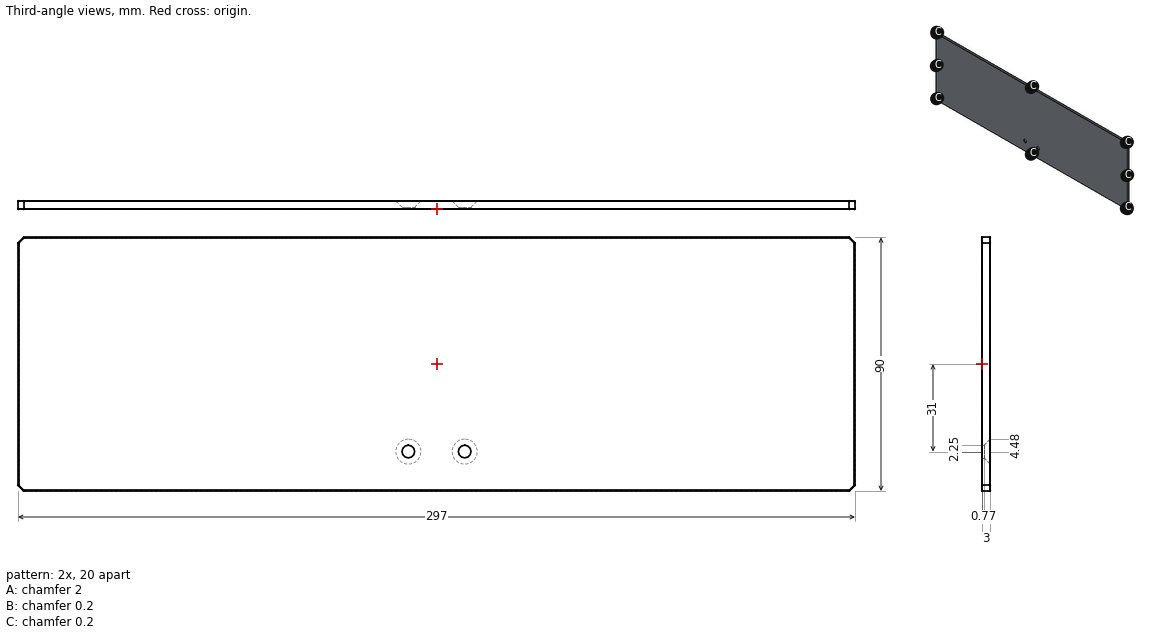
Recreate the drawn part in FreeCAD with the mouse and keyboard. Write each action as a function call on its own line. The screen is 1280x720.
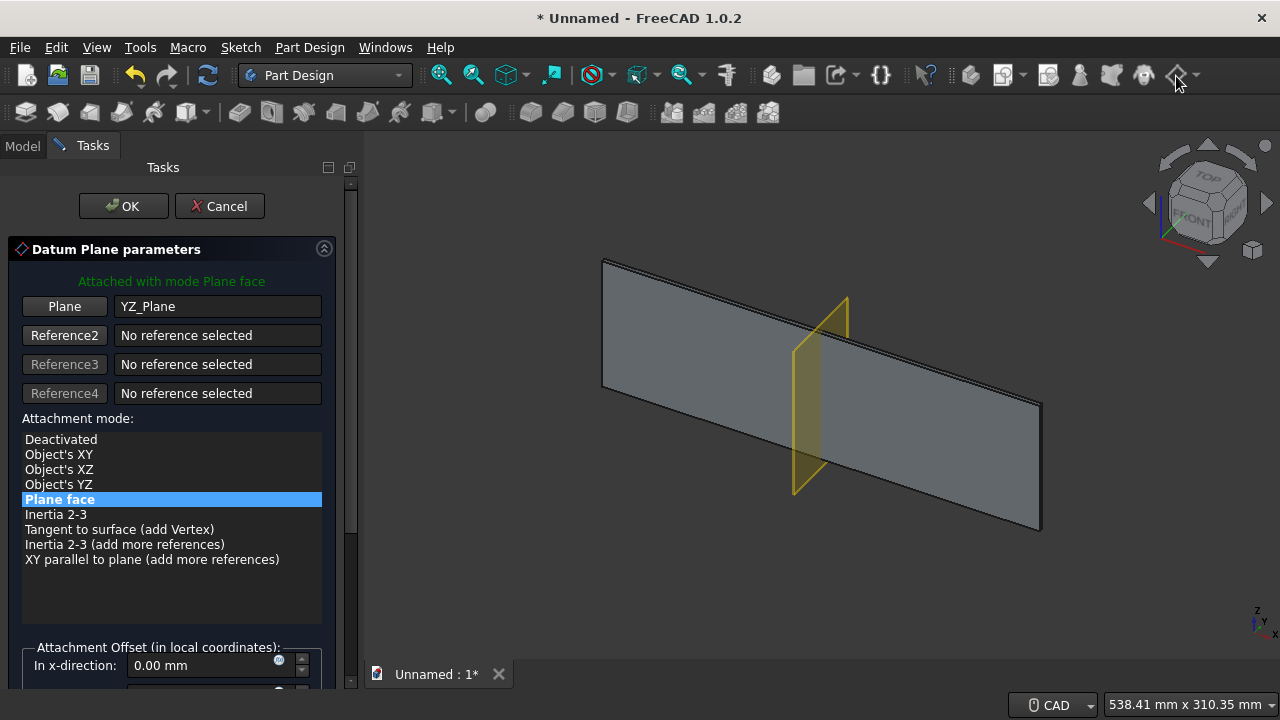
scroll(351, 432, down, 2)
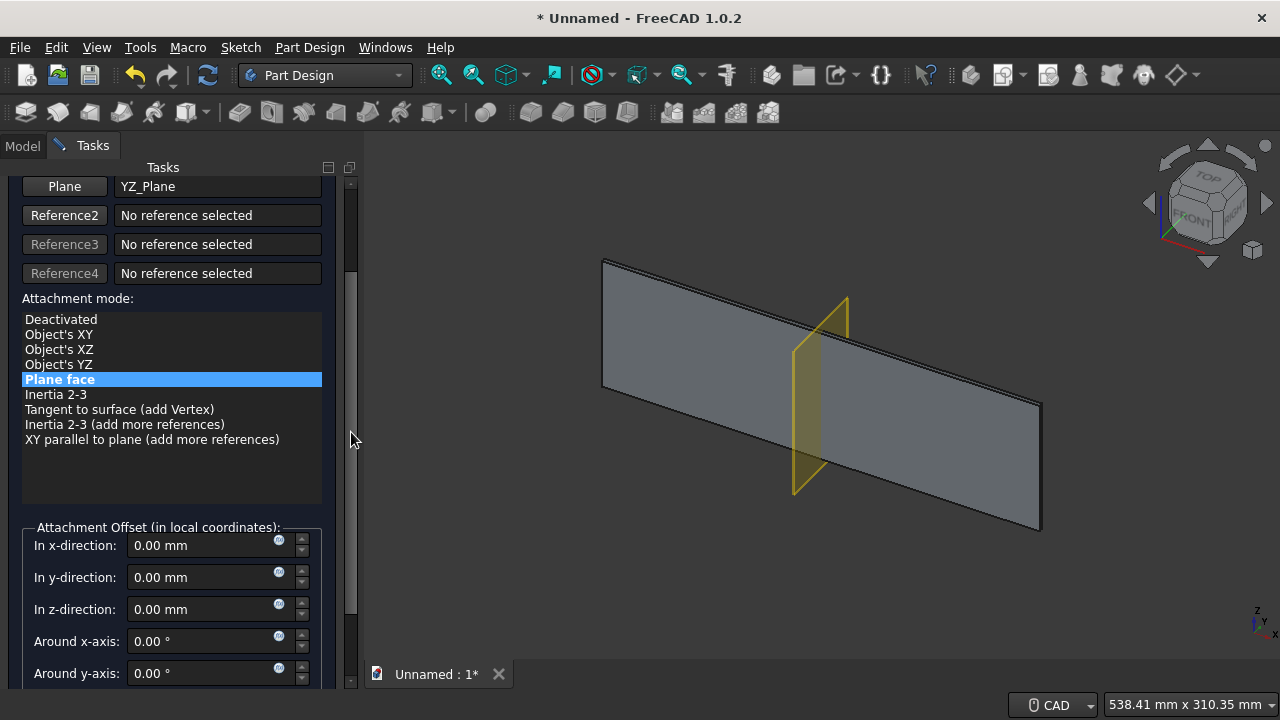
triple_click(210, 609)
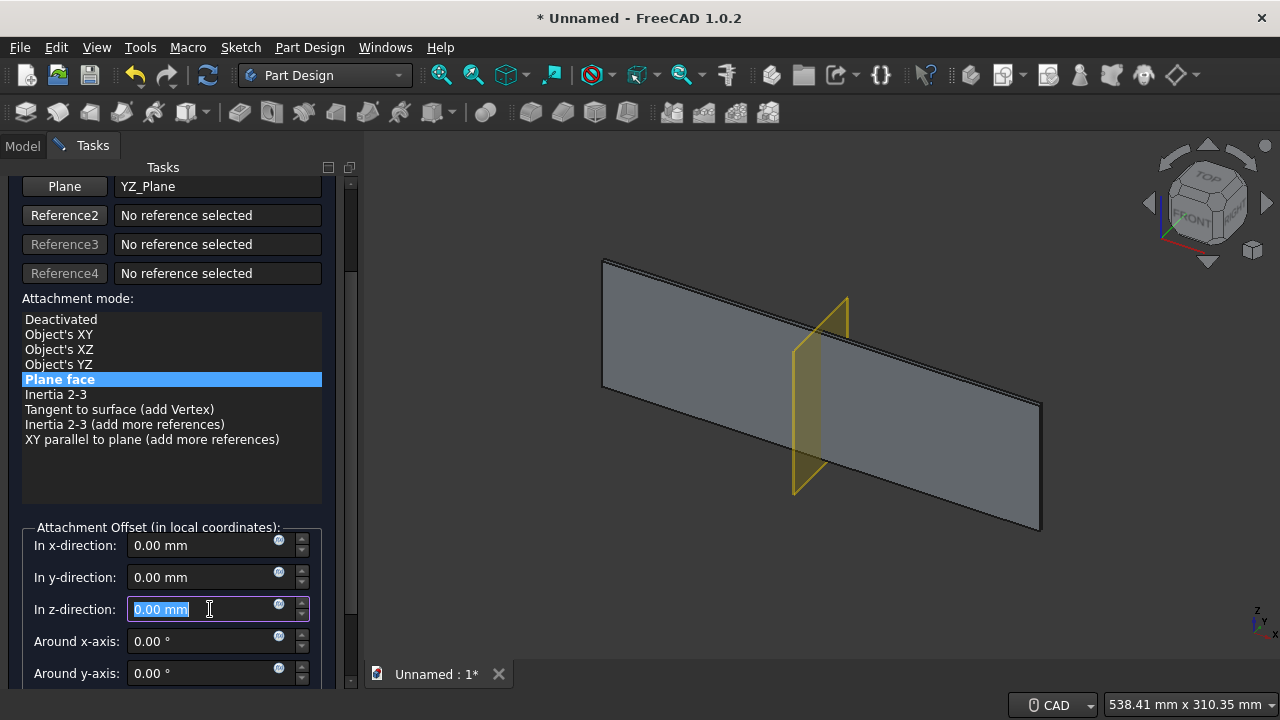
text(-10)
key(Tab)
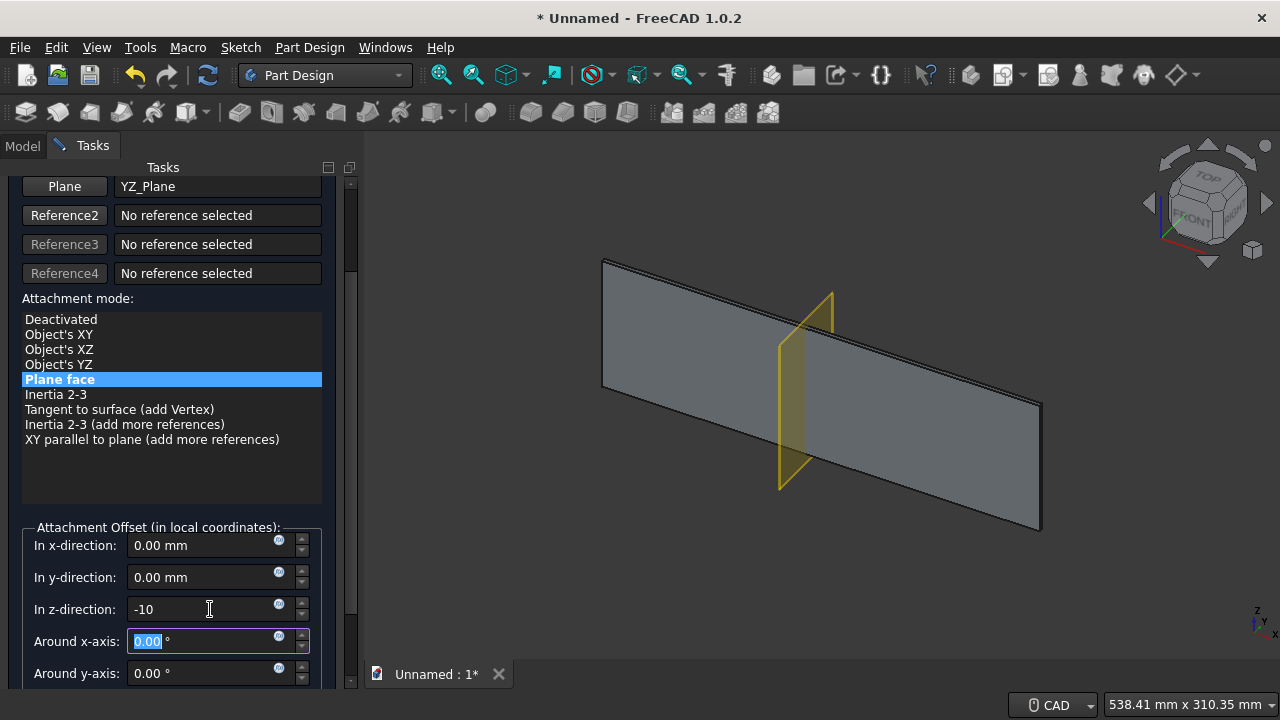
scroll(351, 432, up, 3)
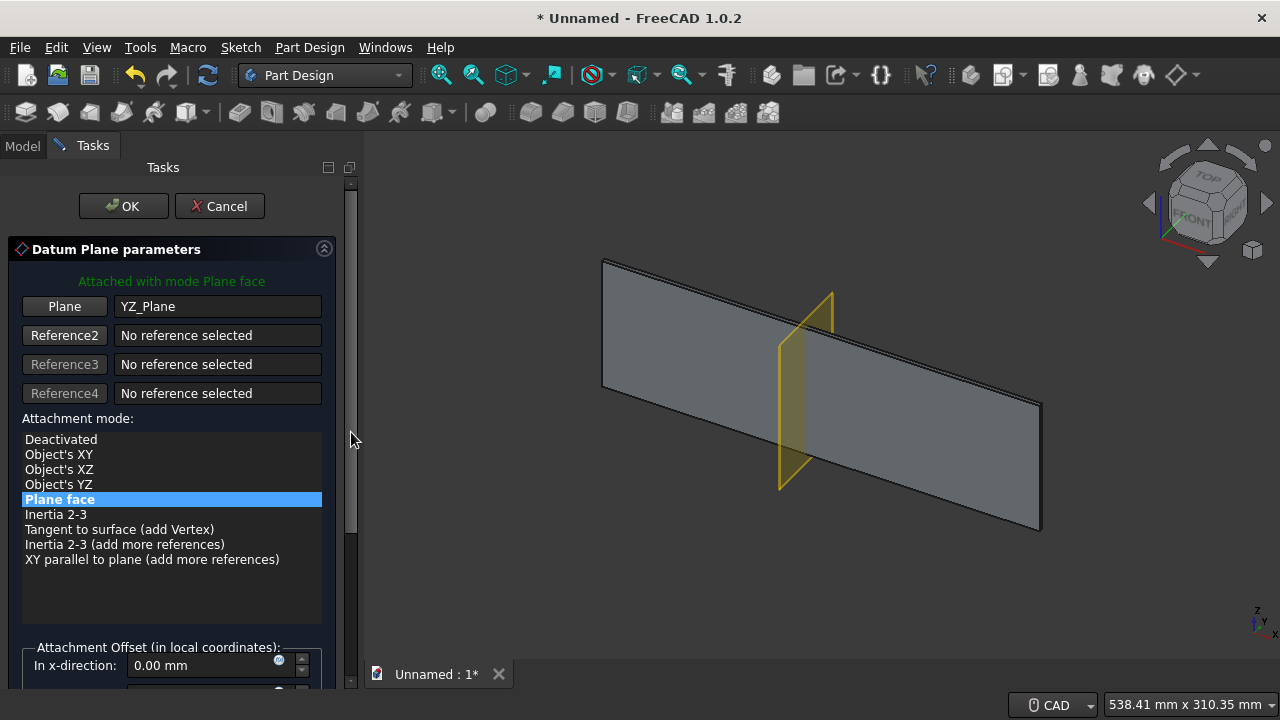
click(124, 206)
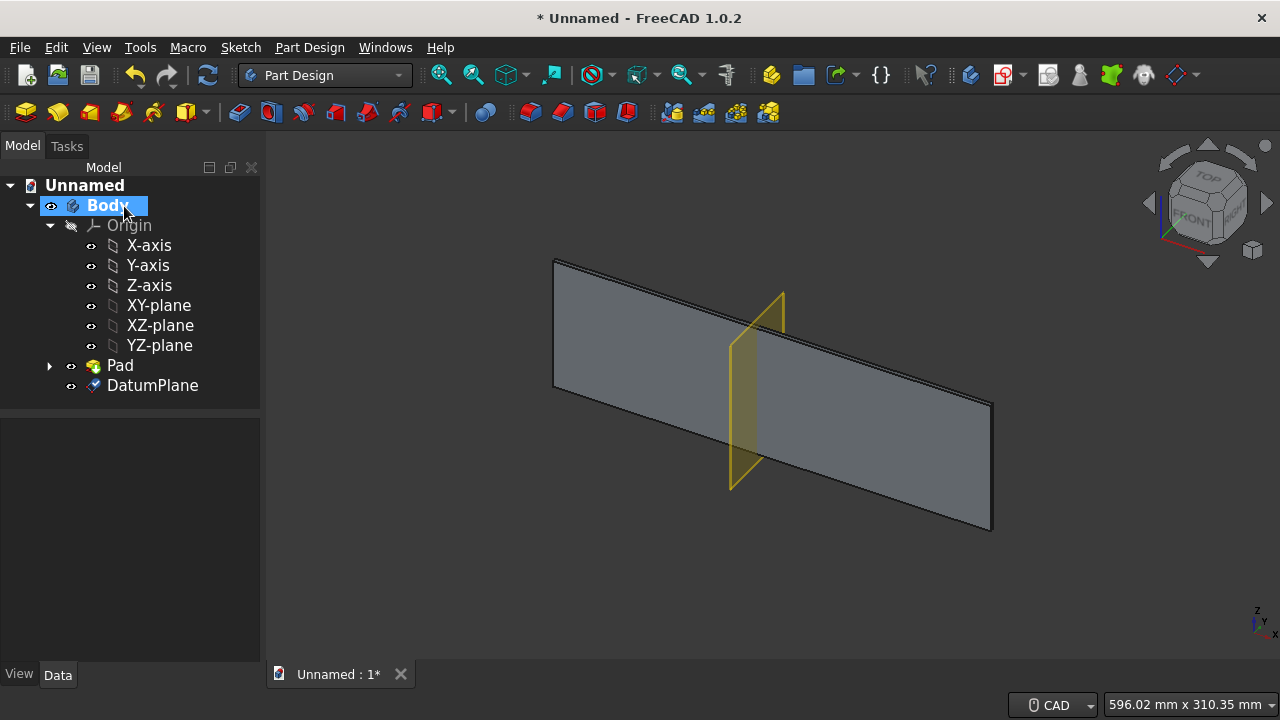
click(116, 386)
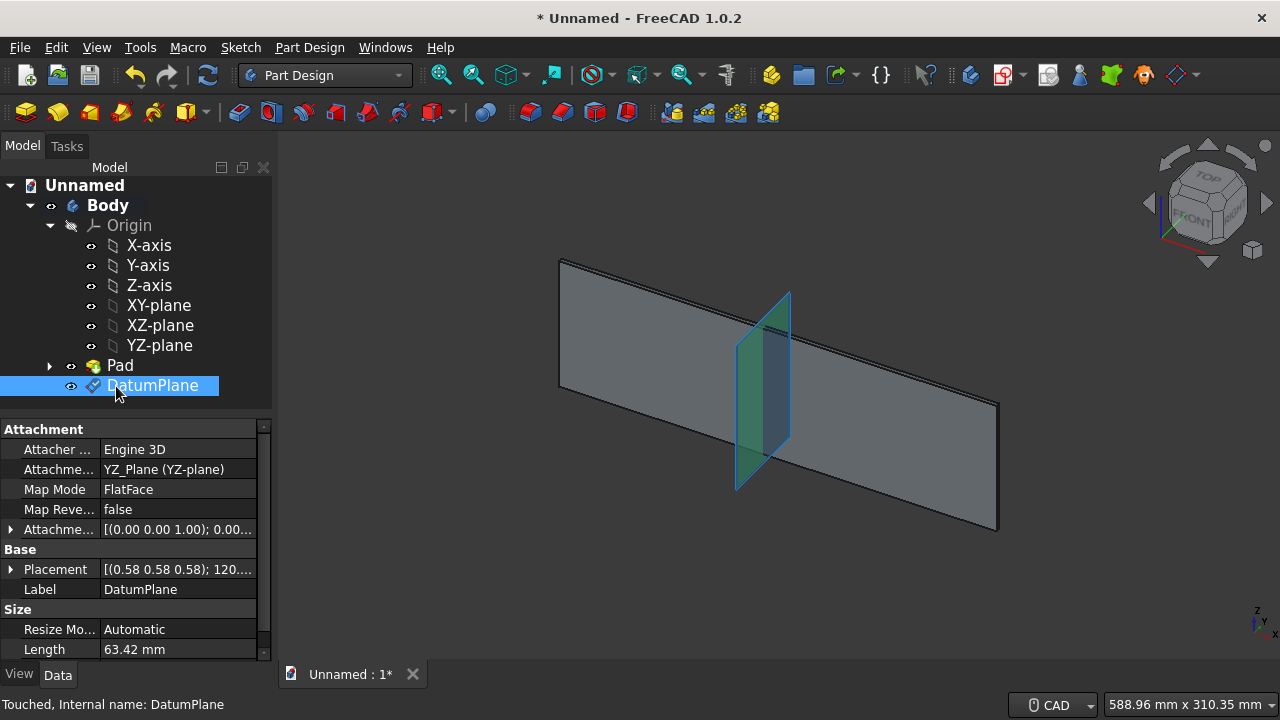
click(1004, 76)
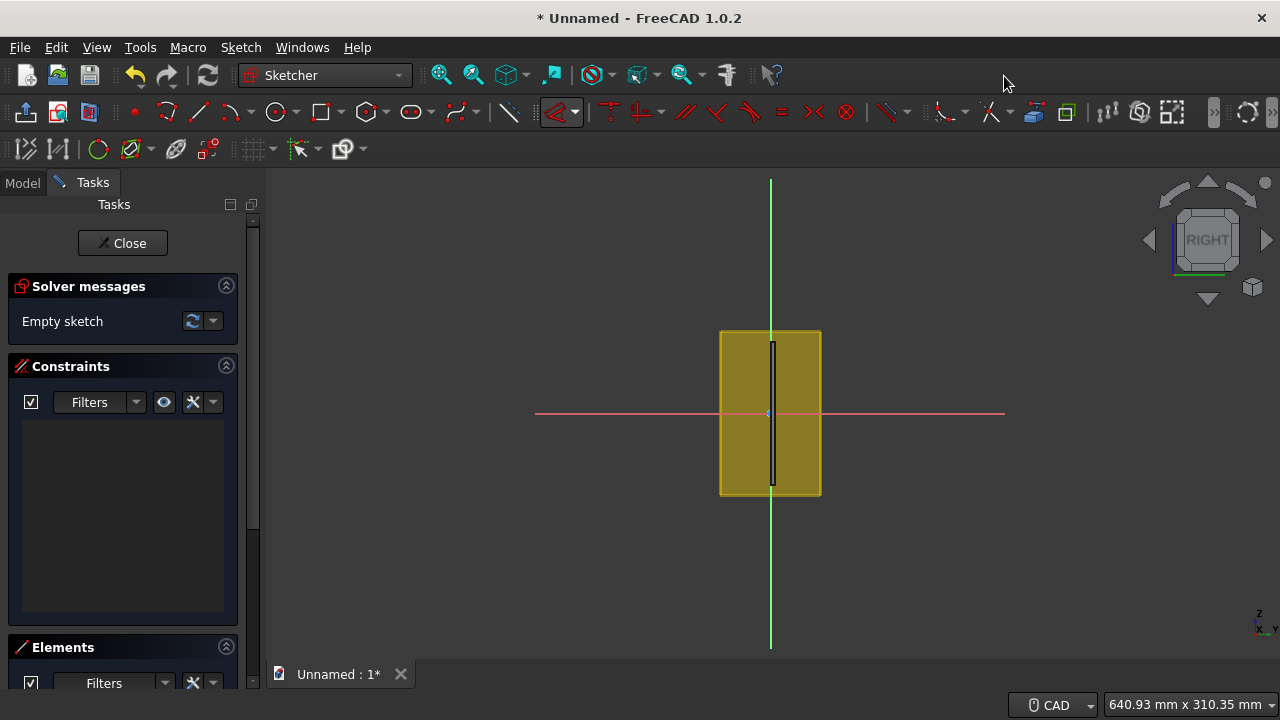
key(q)
key(s)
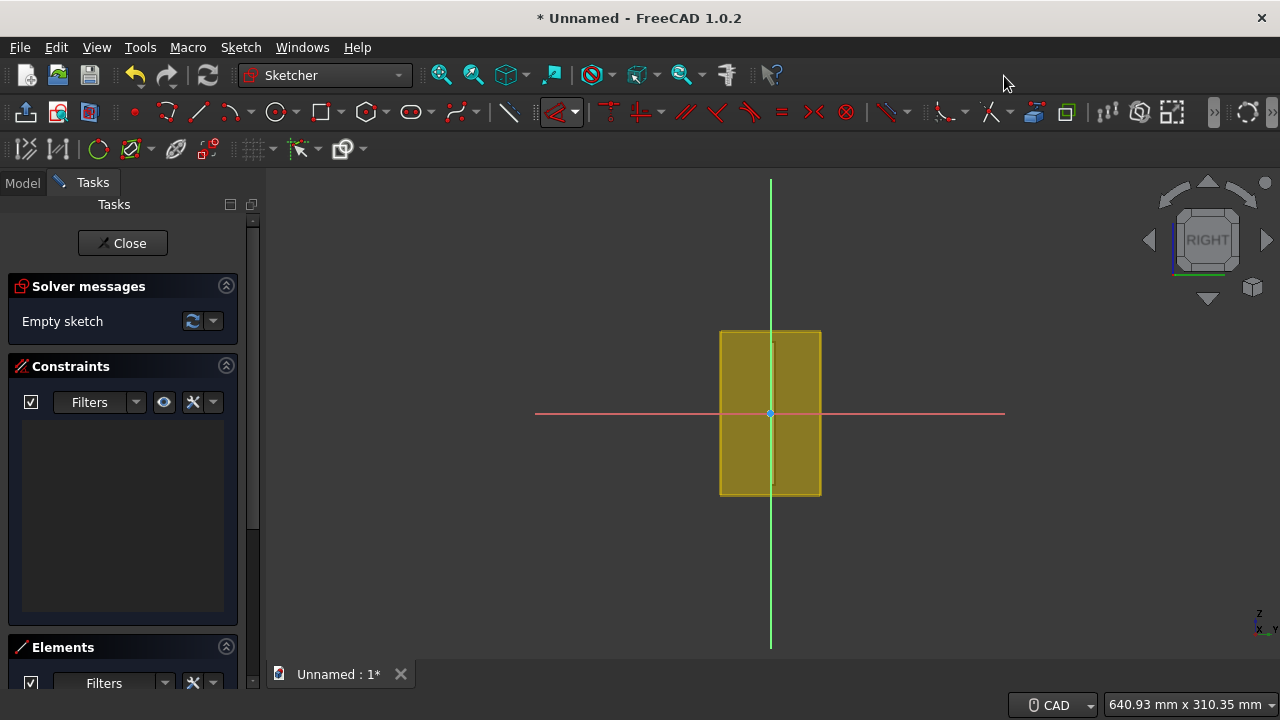
scroll(776, 461, up, 15)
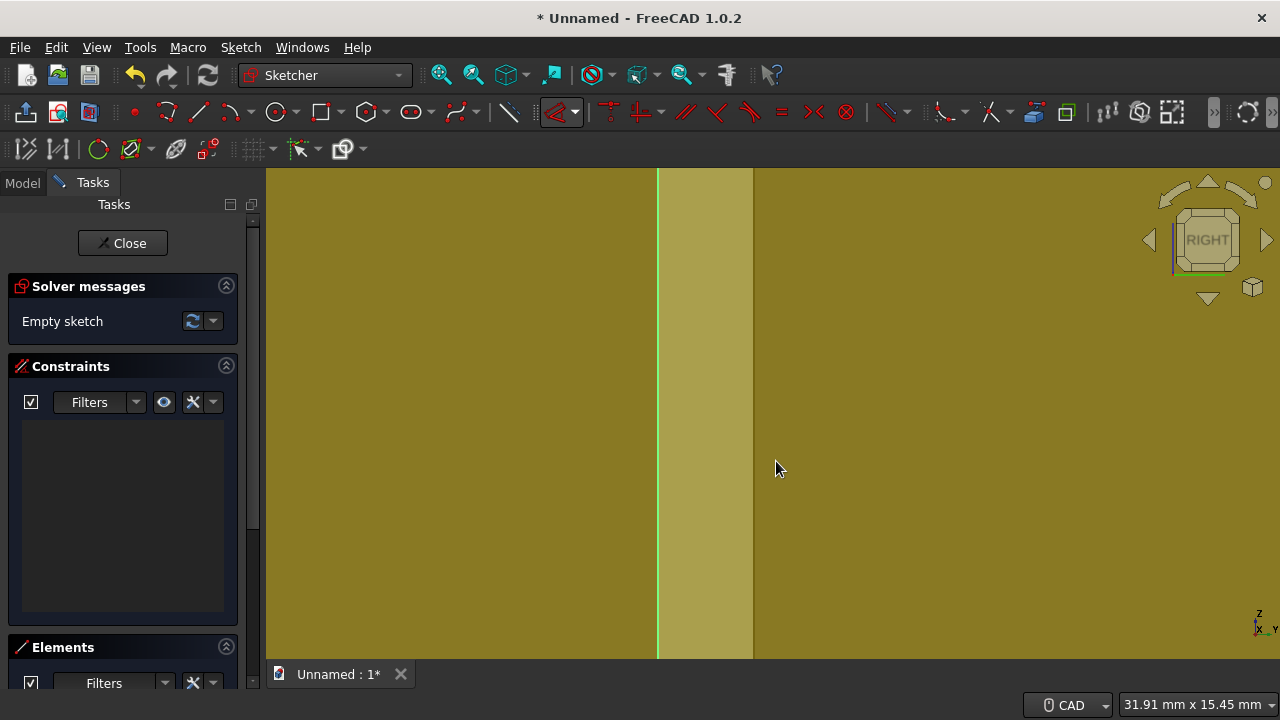
scroll(673, 406, up, 4)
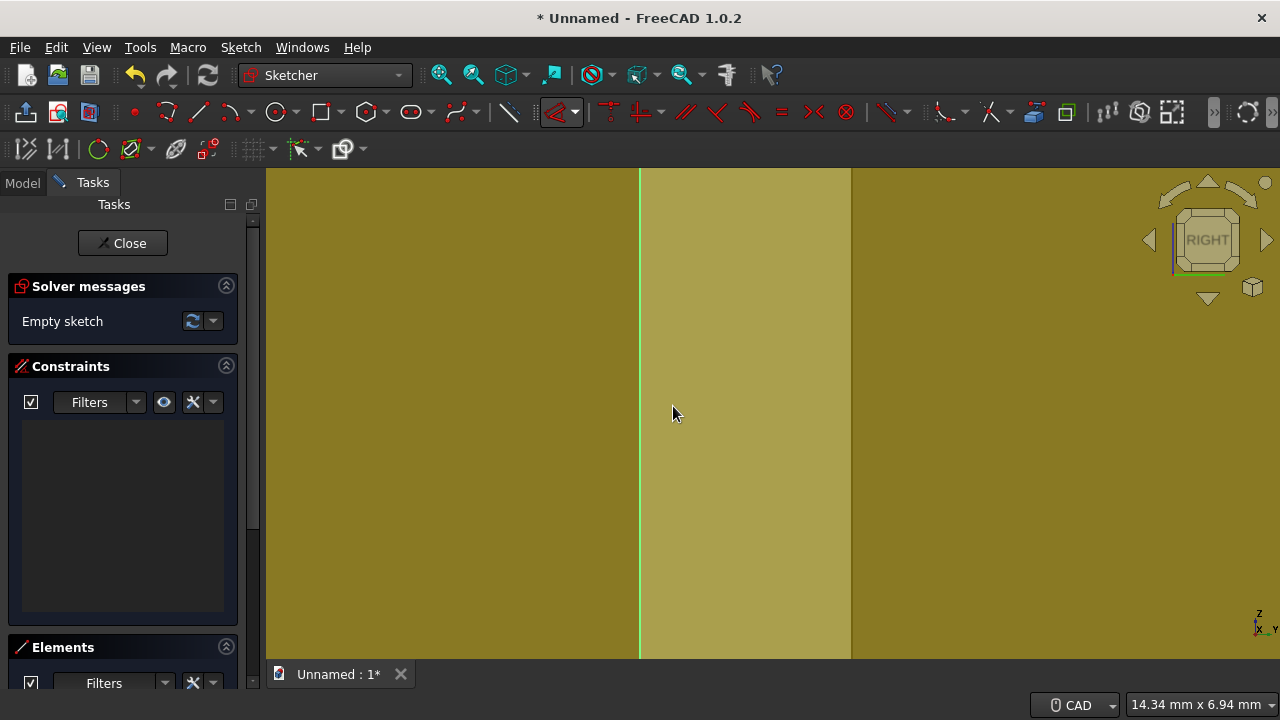
key(g)
key(m)